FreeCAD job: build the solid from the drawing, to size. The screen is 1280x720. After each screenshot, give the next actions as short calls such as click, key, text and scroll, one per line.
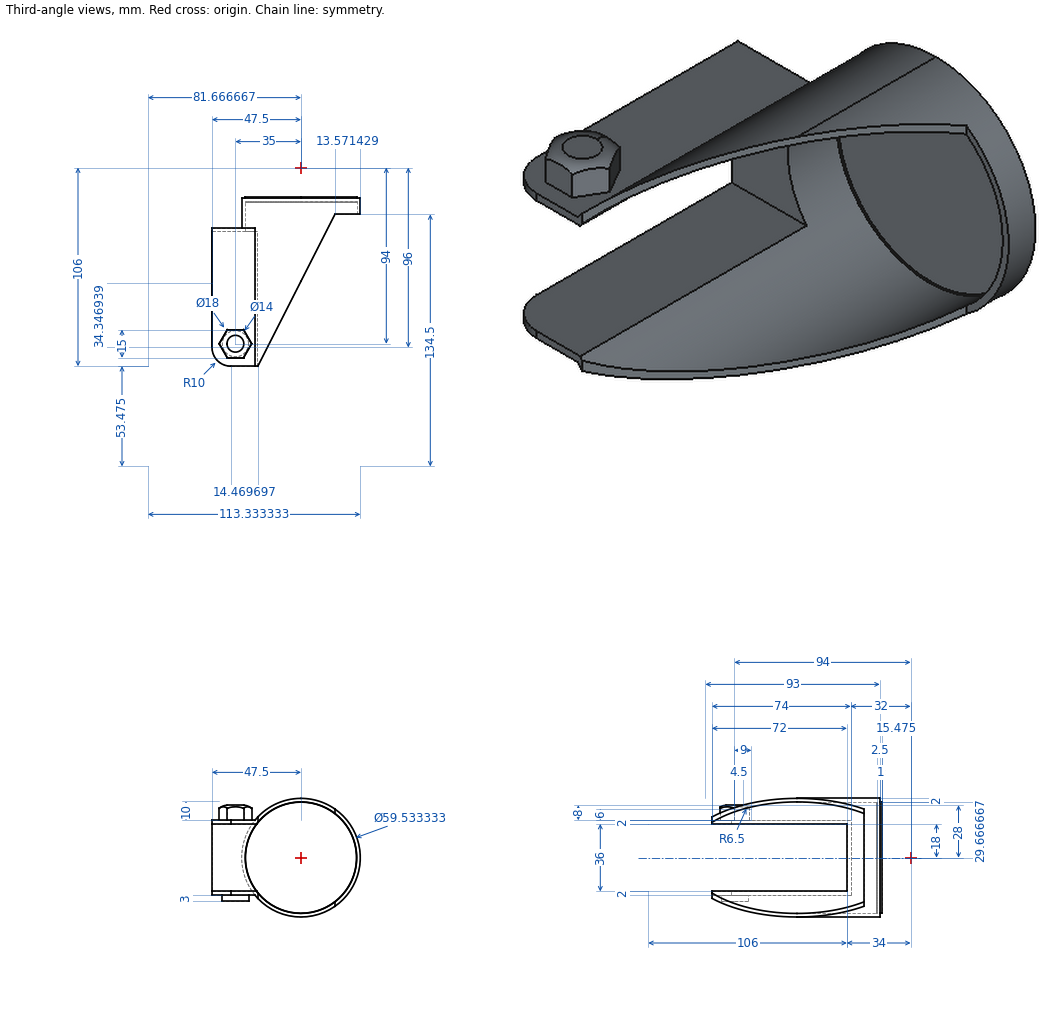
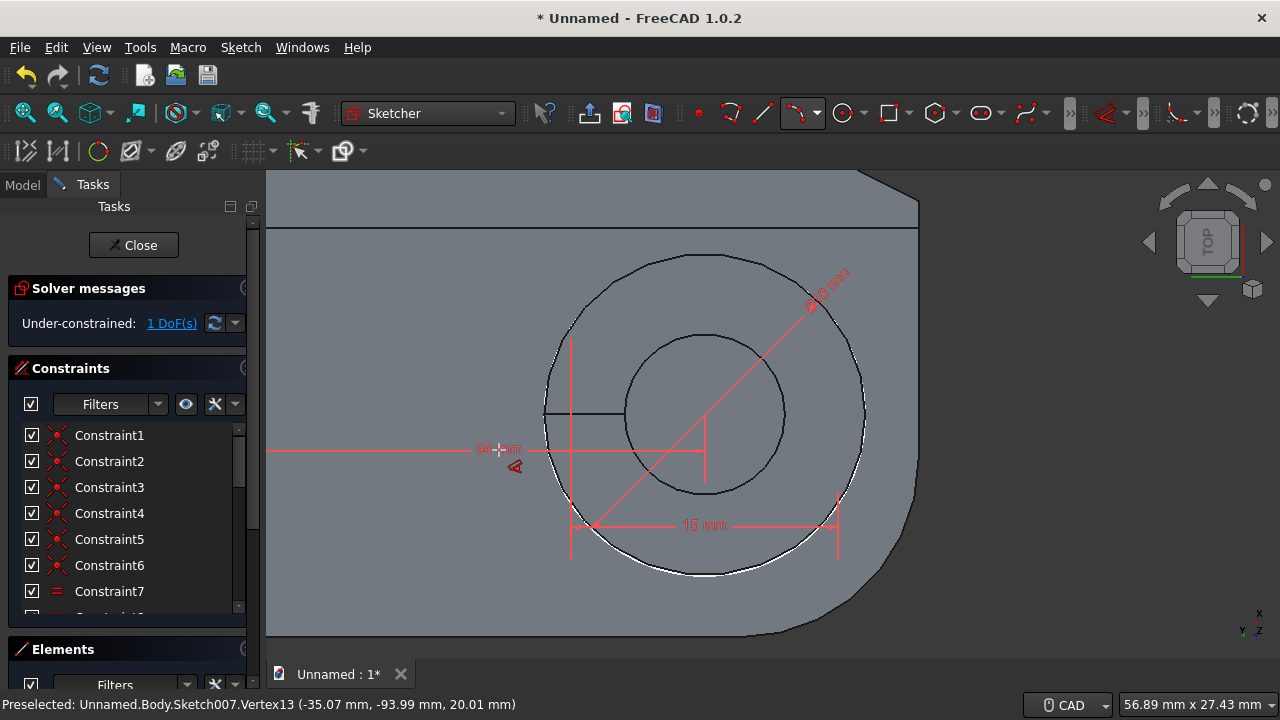
click(705, 416)
click(739, 307)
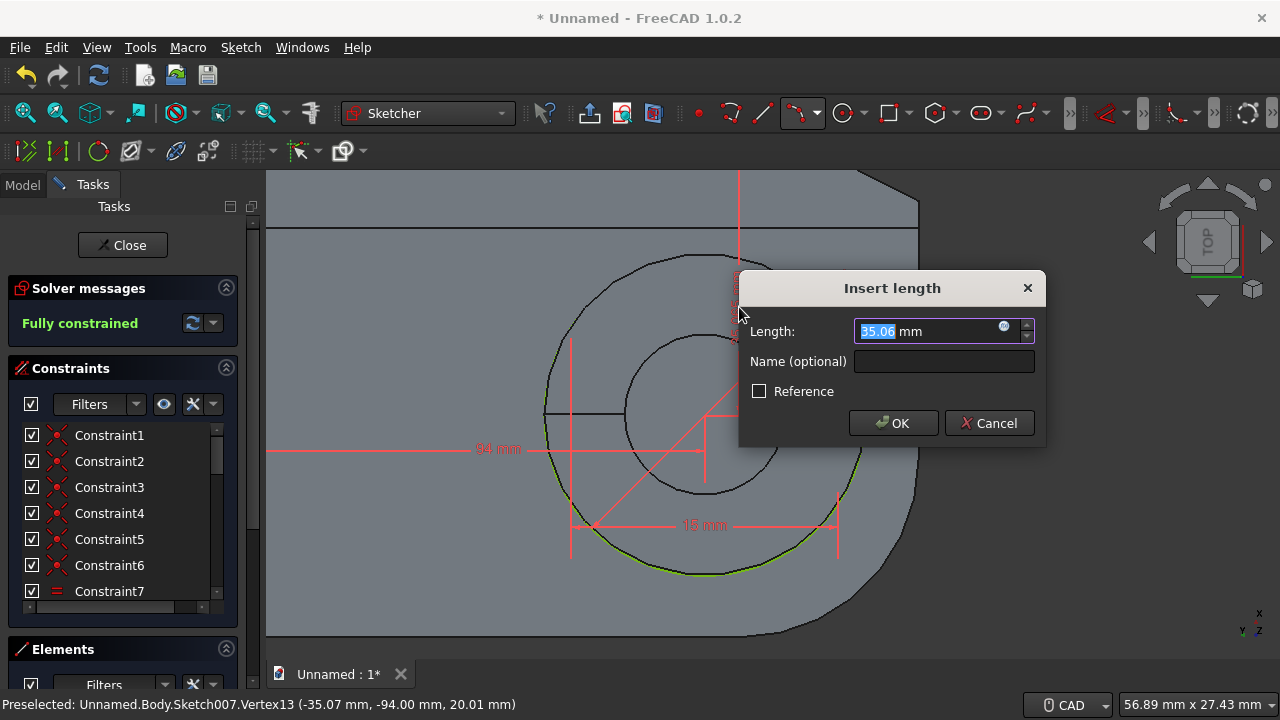
text(35)
key(Return)
key(Escape)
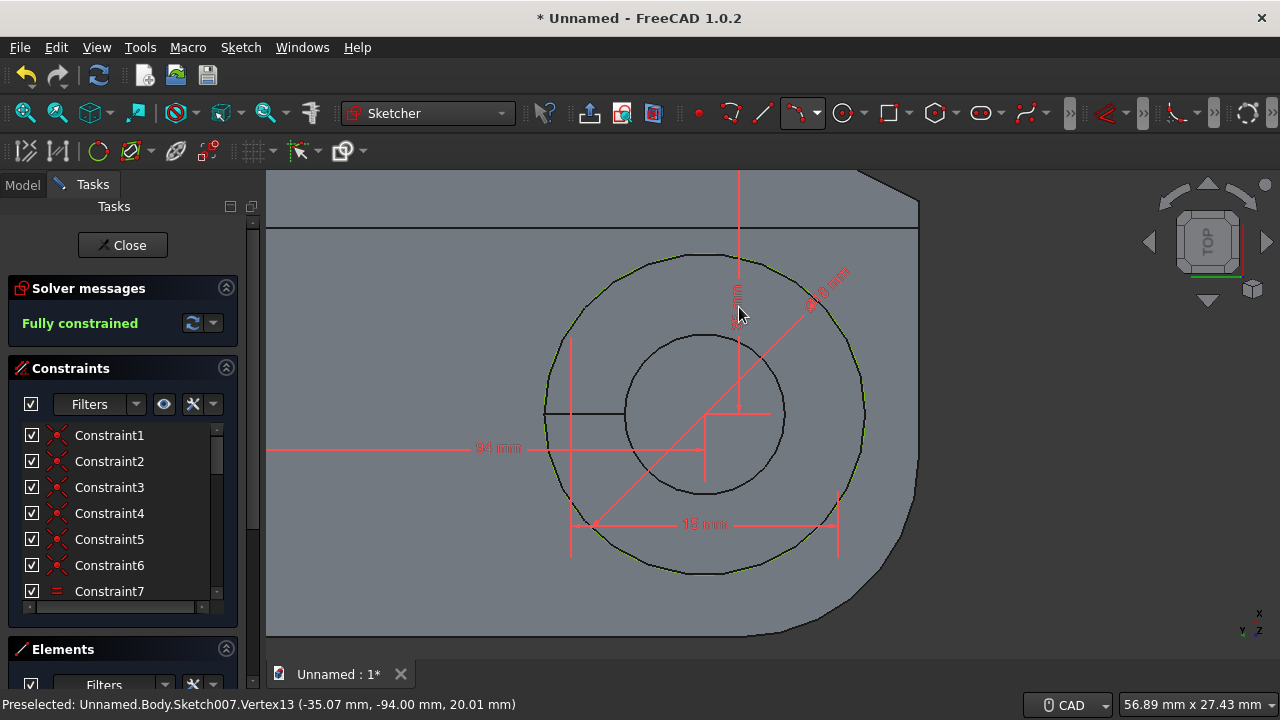
click(123, 245)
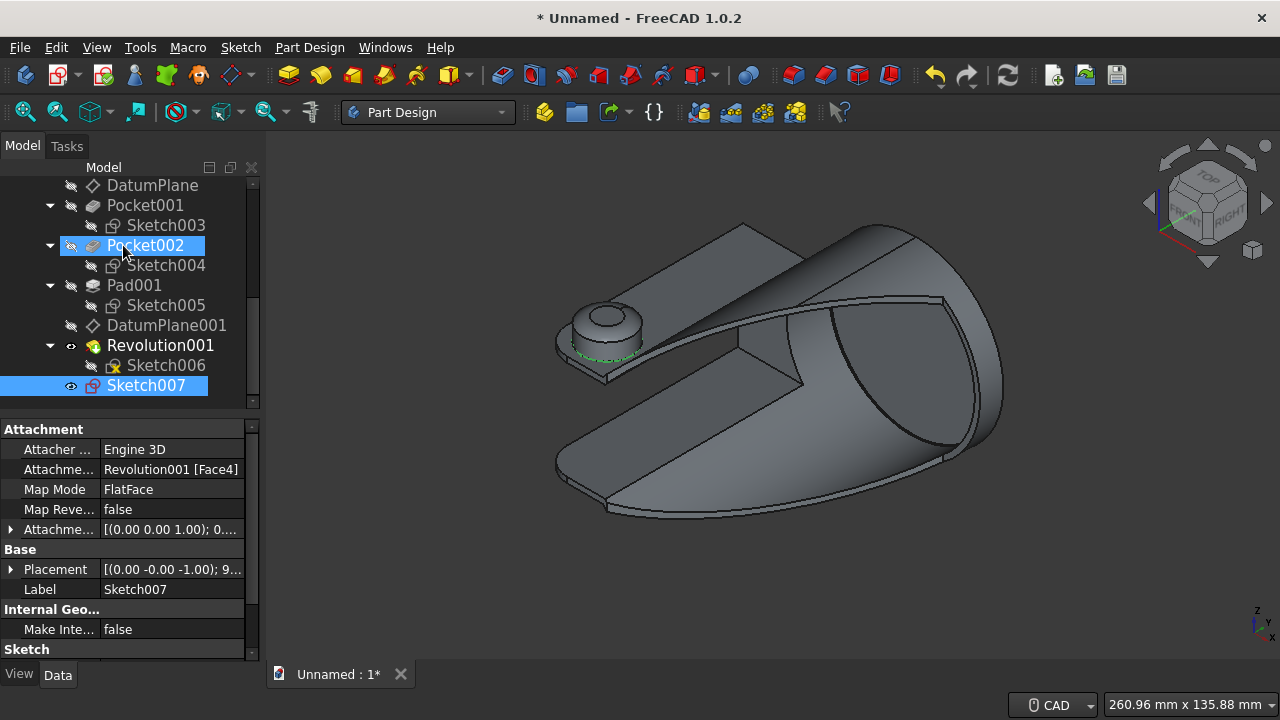
click(504, 76)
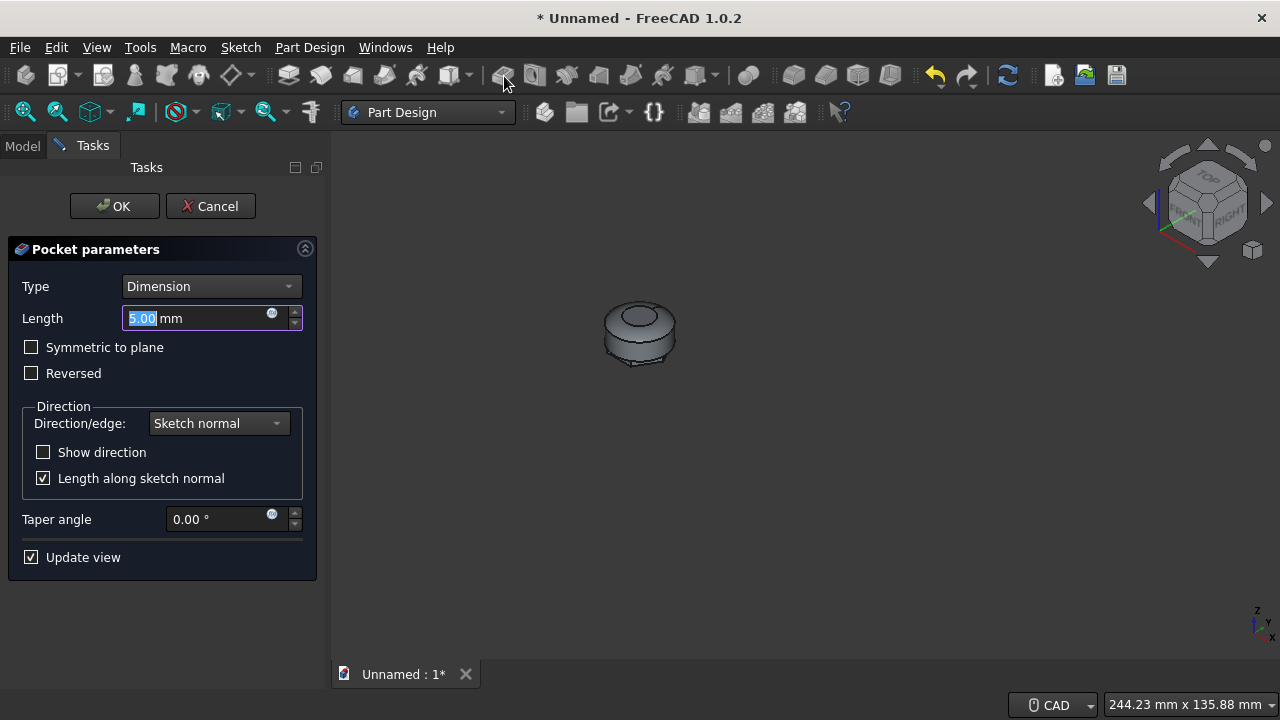
text(10)
key(Tab)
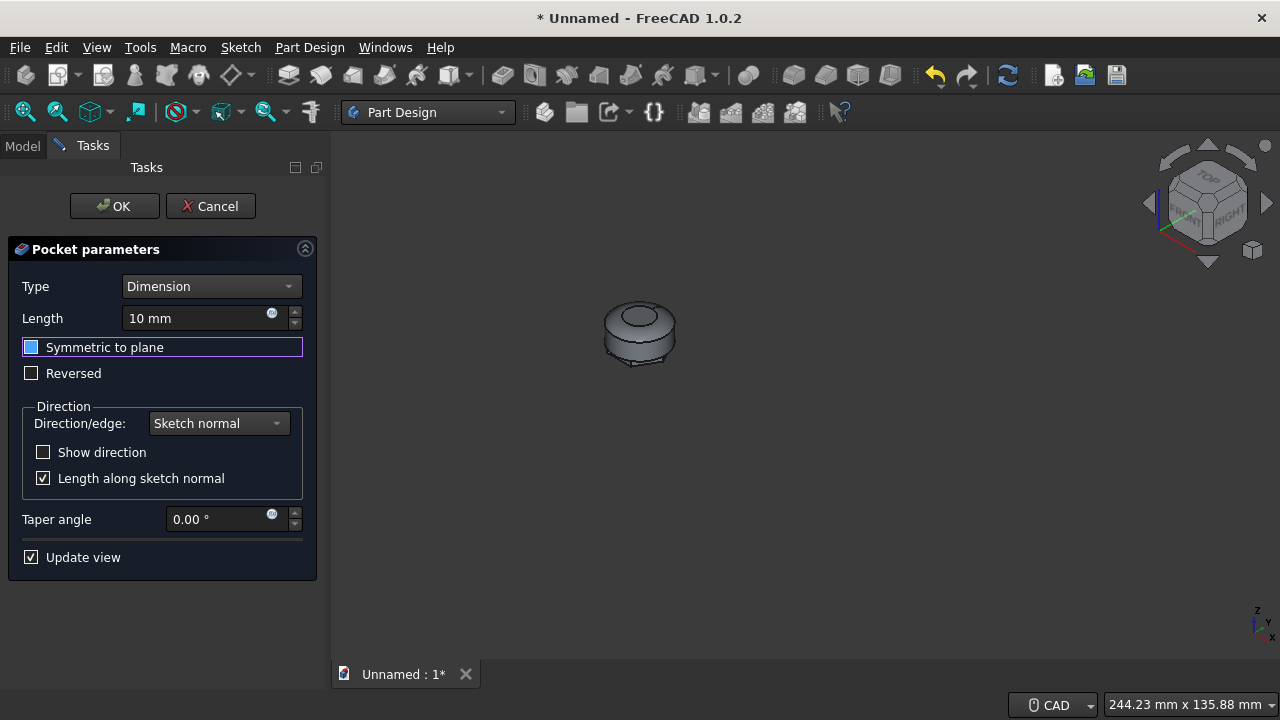
click(30, 373)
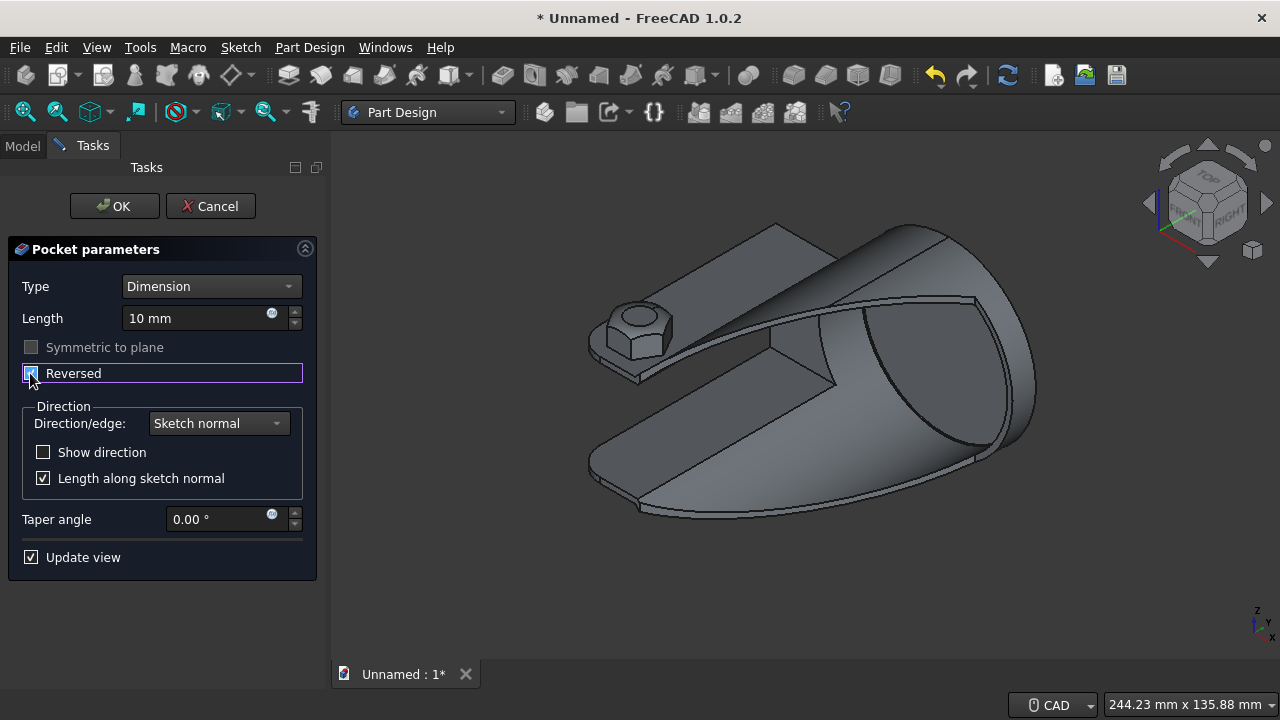
click(115, 206)